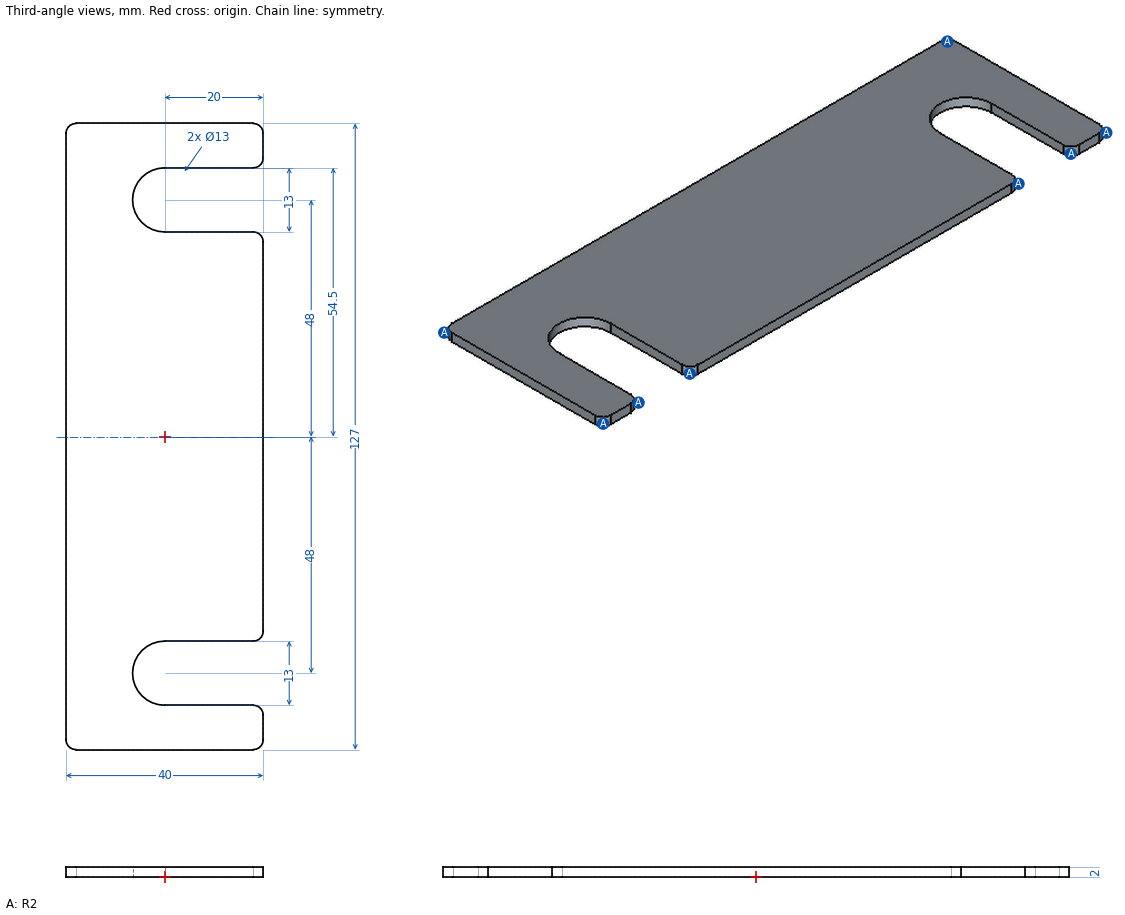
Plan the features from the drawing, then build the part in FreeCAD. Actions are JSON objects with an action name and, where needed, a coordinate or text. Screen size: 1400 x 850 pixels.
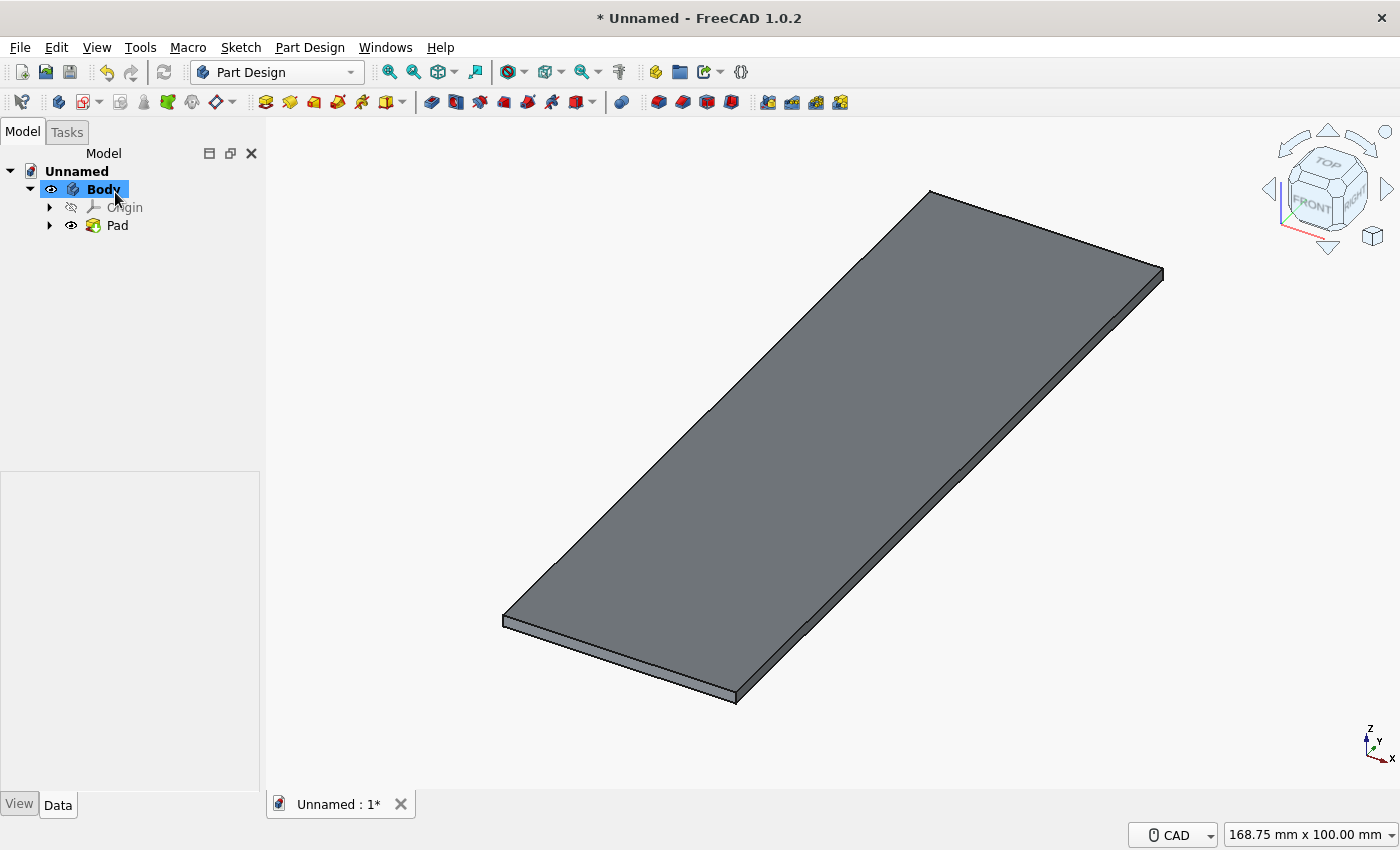
{"action": "left_click", "coordinate": [955, 320]}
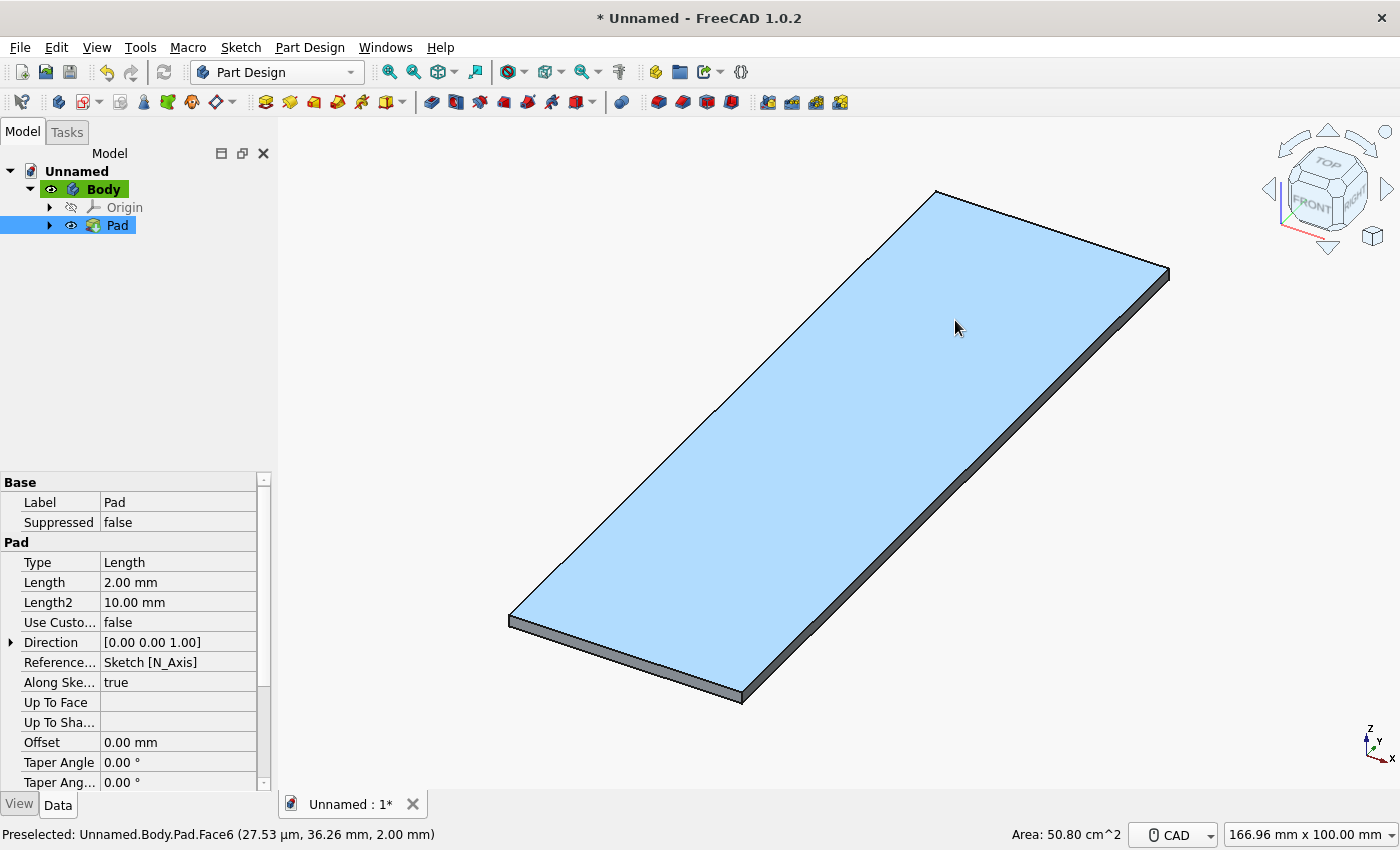
{"action": "left_click", "coordinate": [84, 102]}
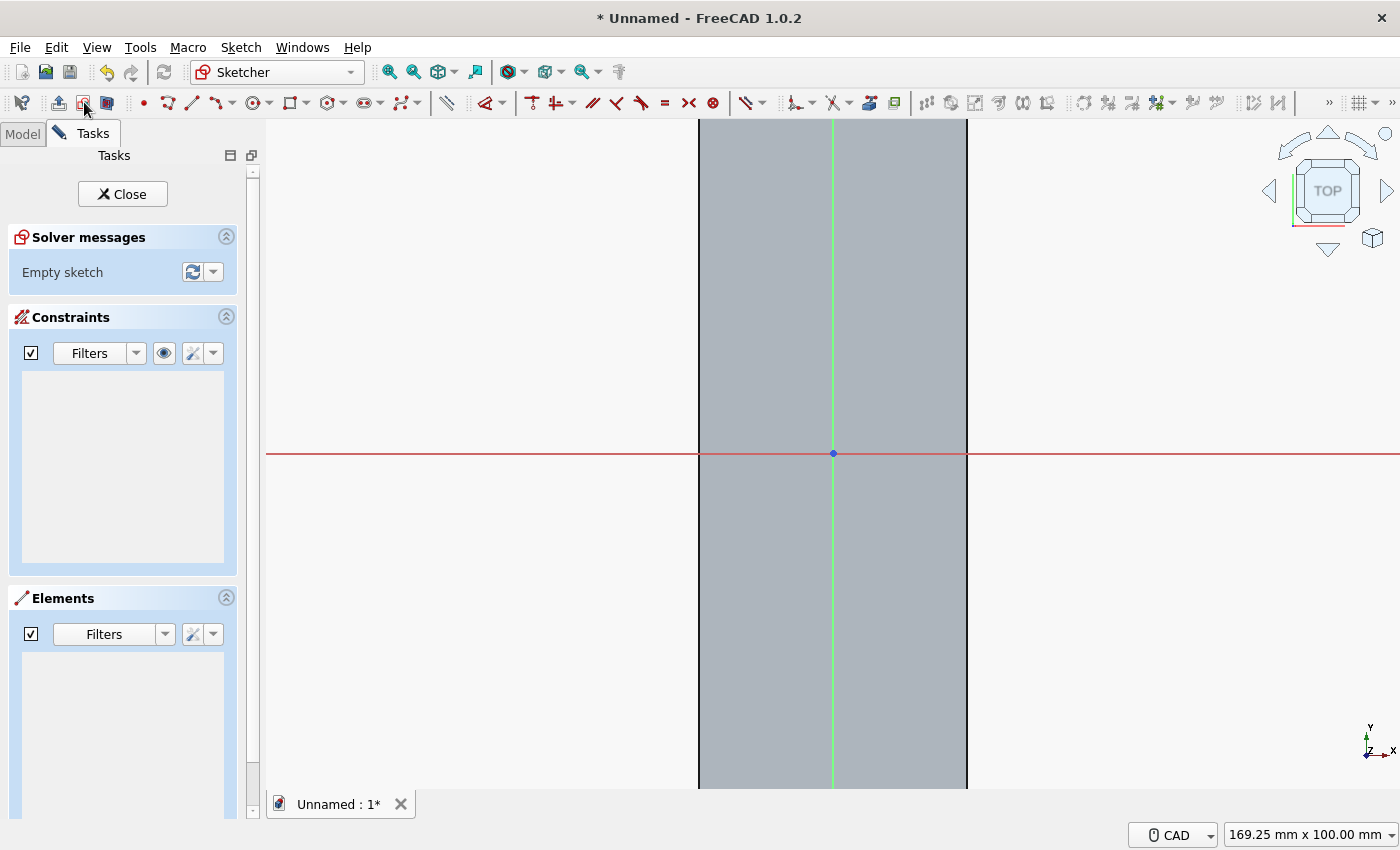
{"action": "scroll", "coordinate": [681, 454], "scroll_direction": "down", "scroll_amount": 3}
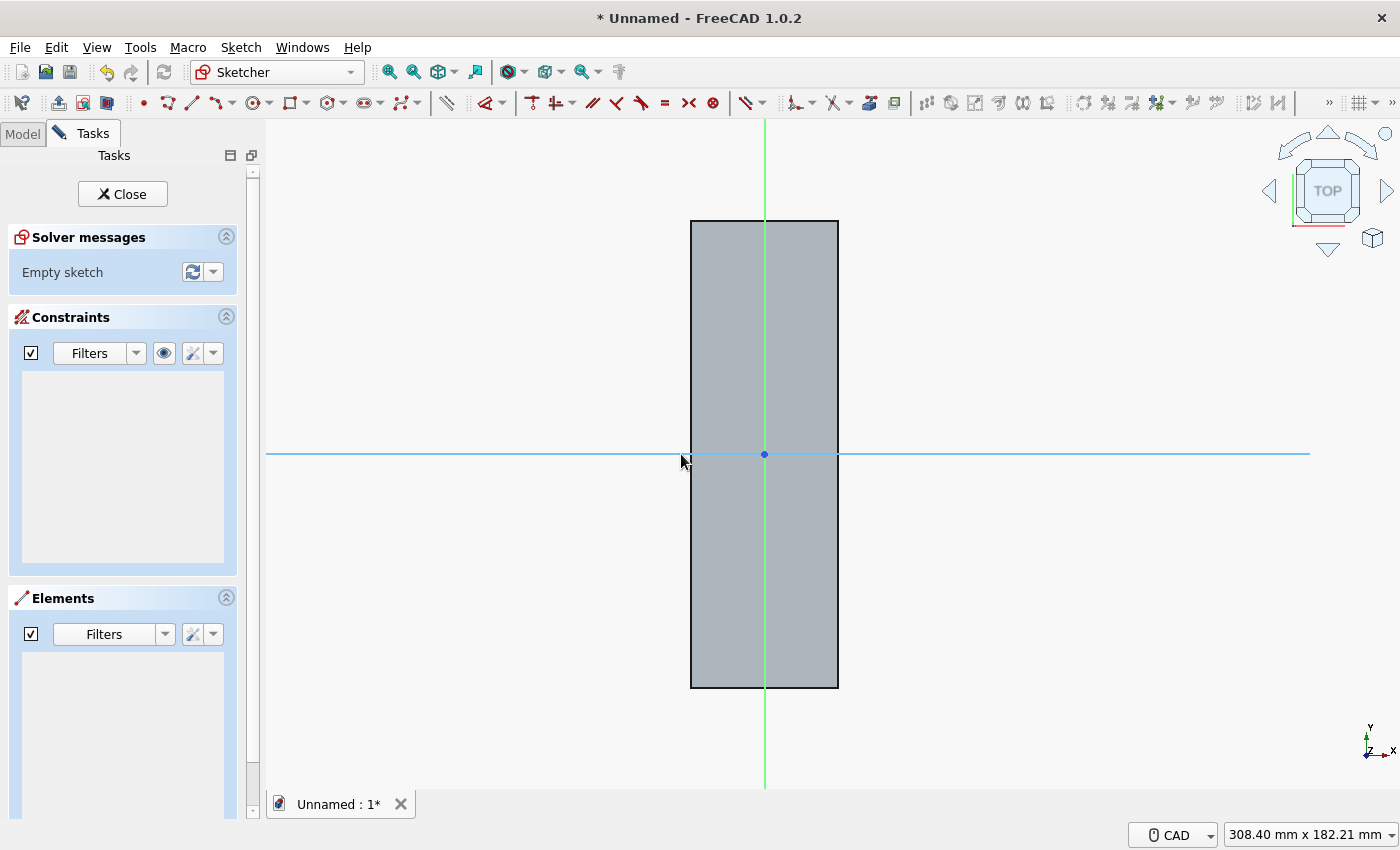
{"action": "left_click", "coordinate": [254, 104]}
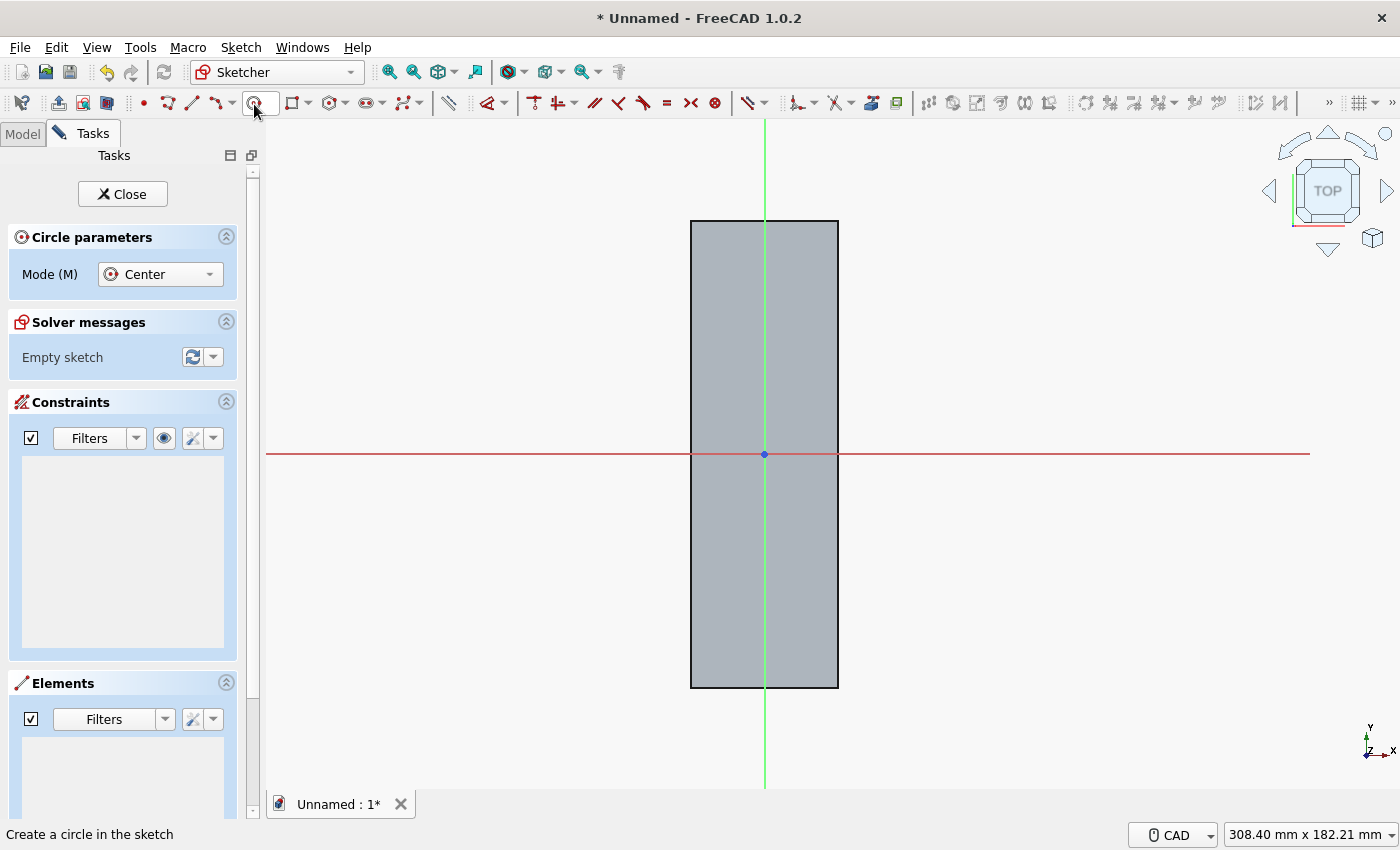
{"action": "left_click", "coordinate": [765, 278]}
{"action": "left_click", "coordinate": [781, 261]}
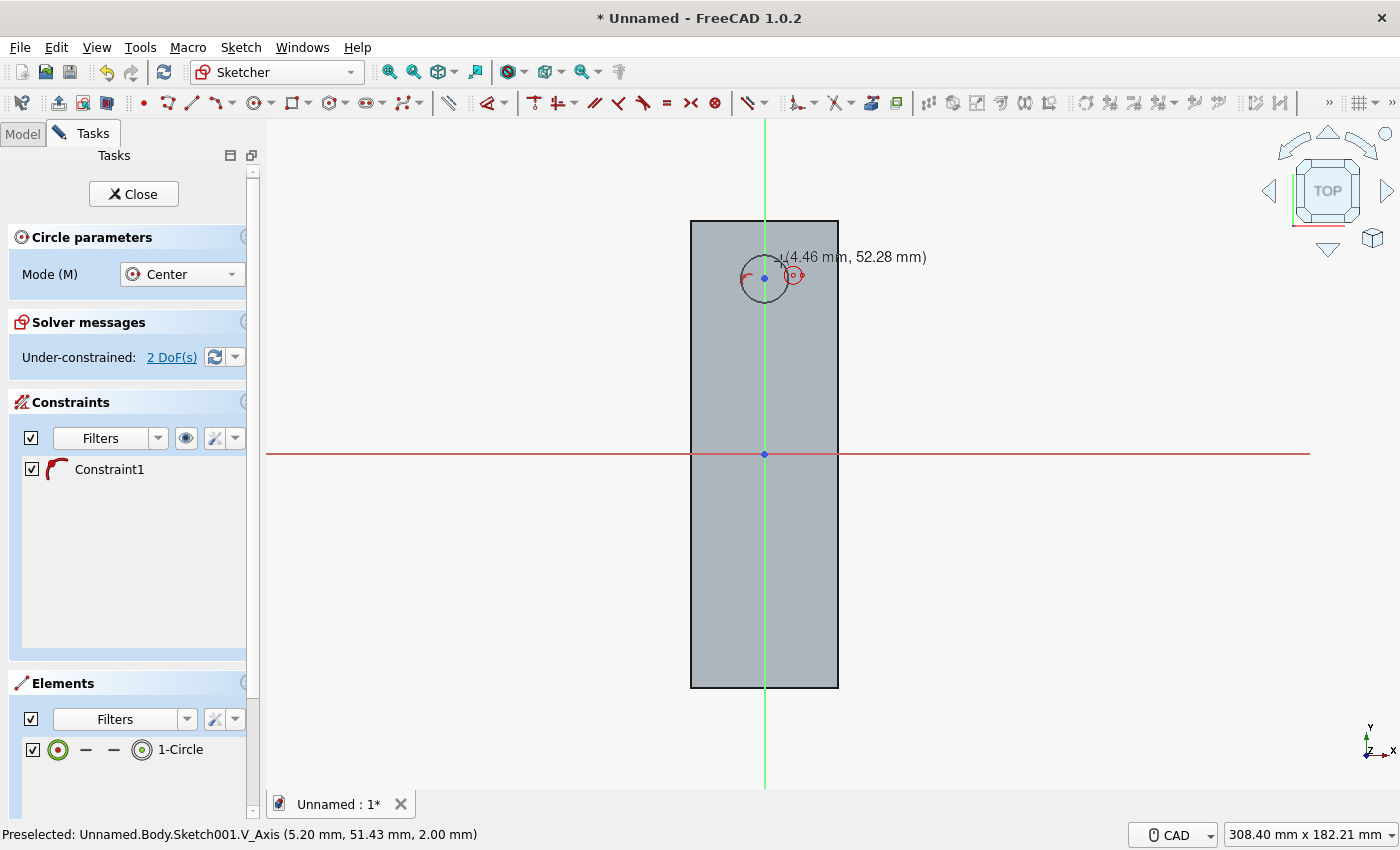
{"action": "left_click", "coordinate": [765, 631]}
{"action": "left_click", "coordinate": [781, 614]}
{"action": "key", "text": "Escape"}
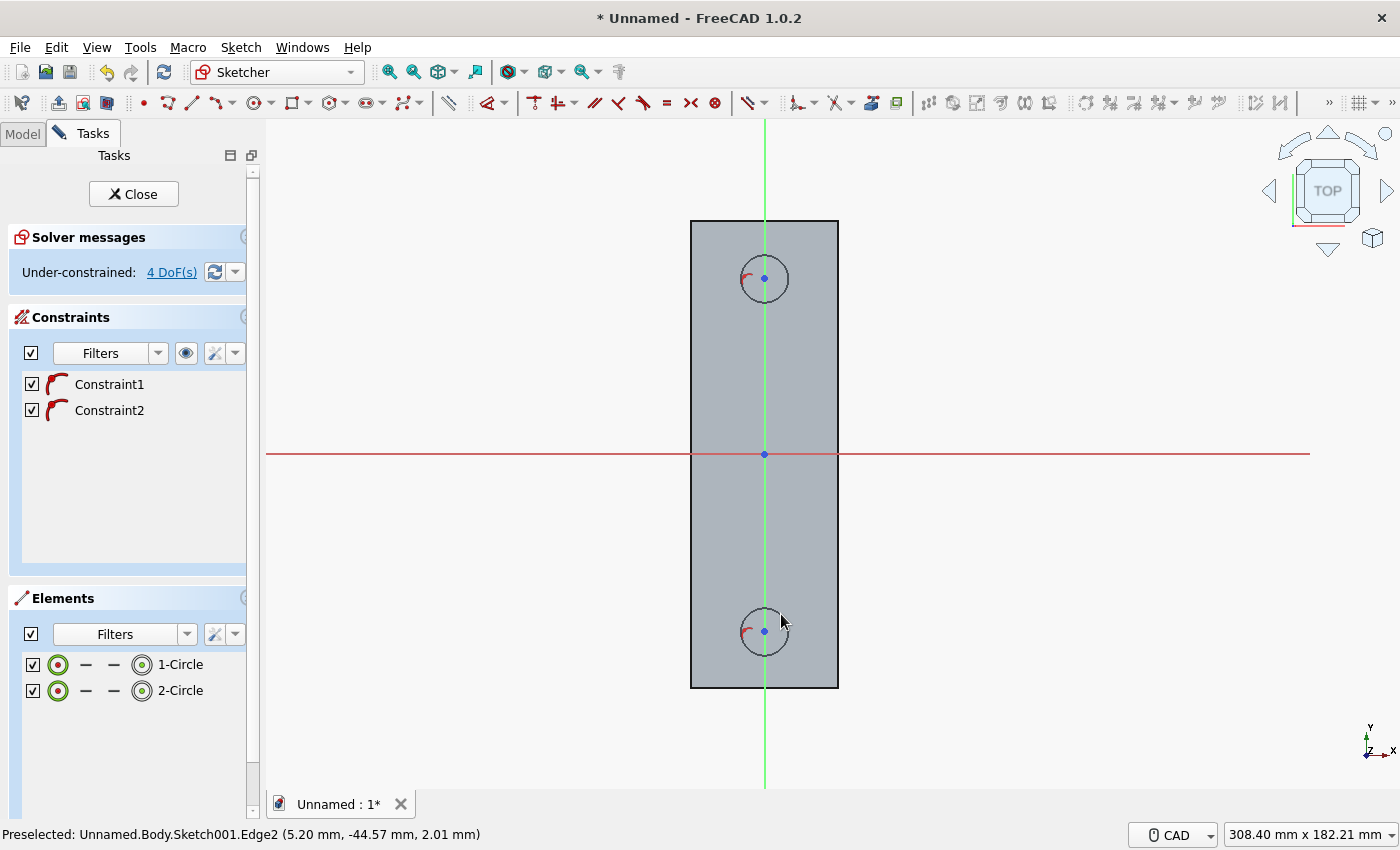
{"action": "left_click", "coordinate": [781, 262]}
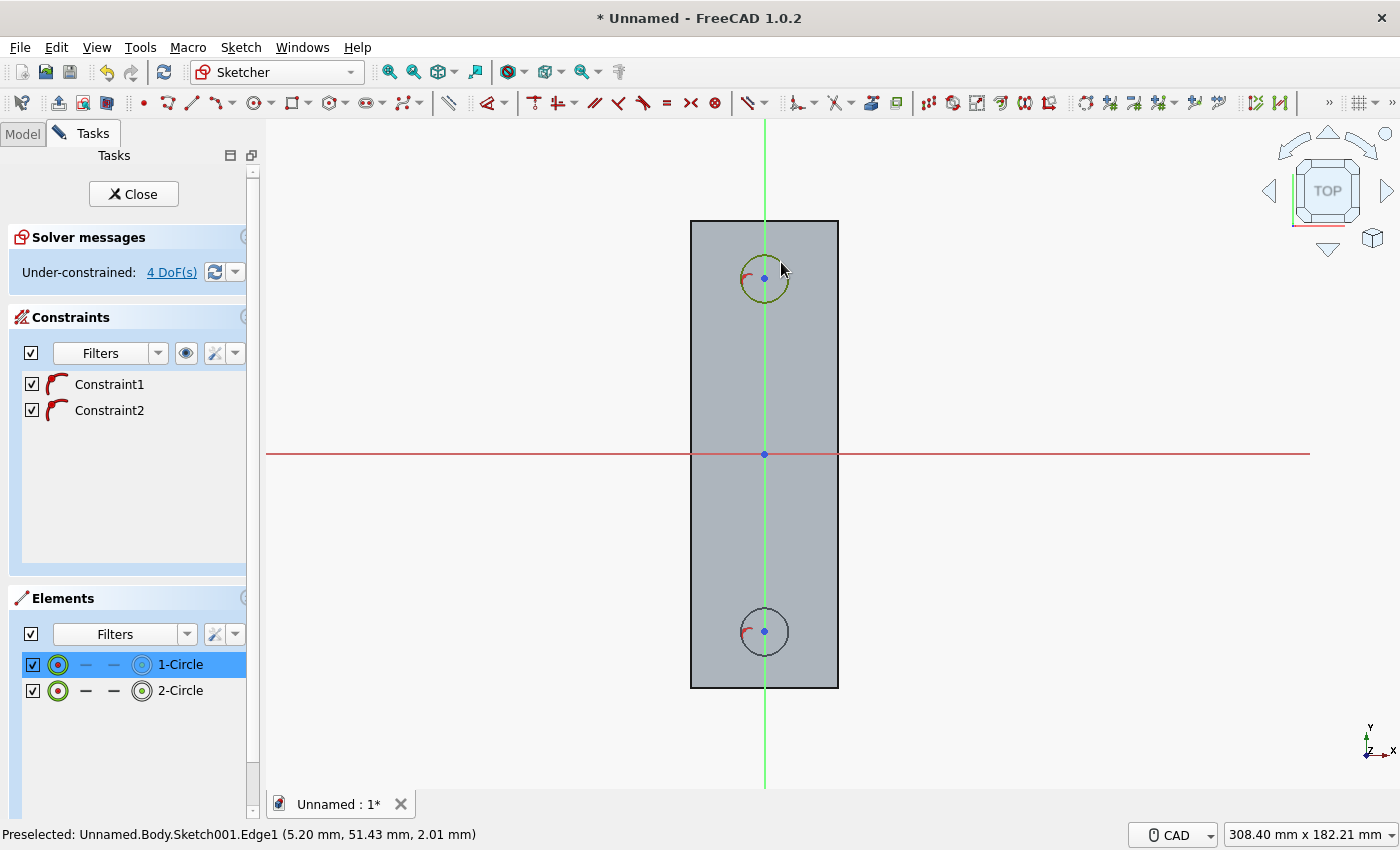
{"action": "left_click", "coordinate": [781, 615]}